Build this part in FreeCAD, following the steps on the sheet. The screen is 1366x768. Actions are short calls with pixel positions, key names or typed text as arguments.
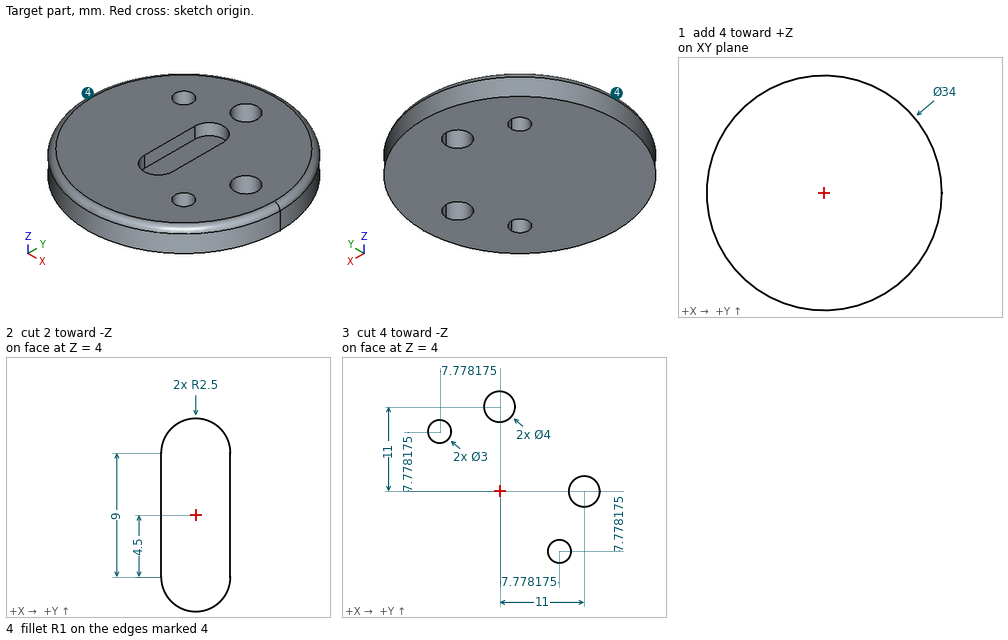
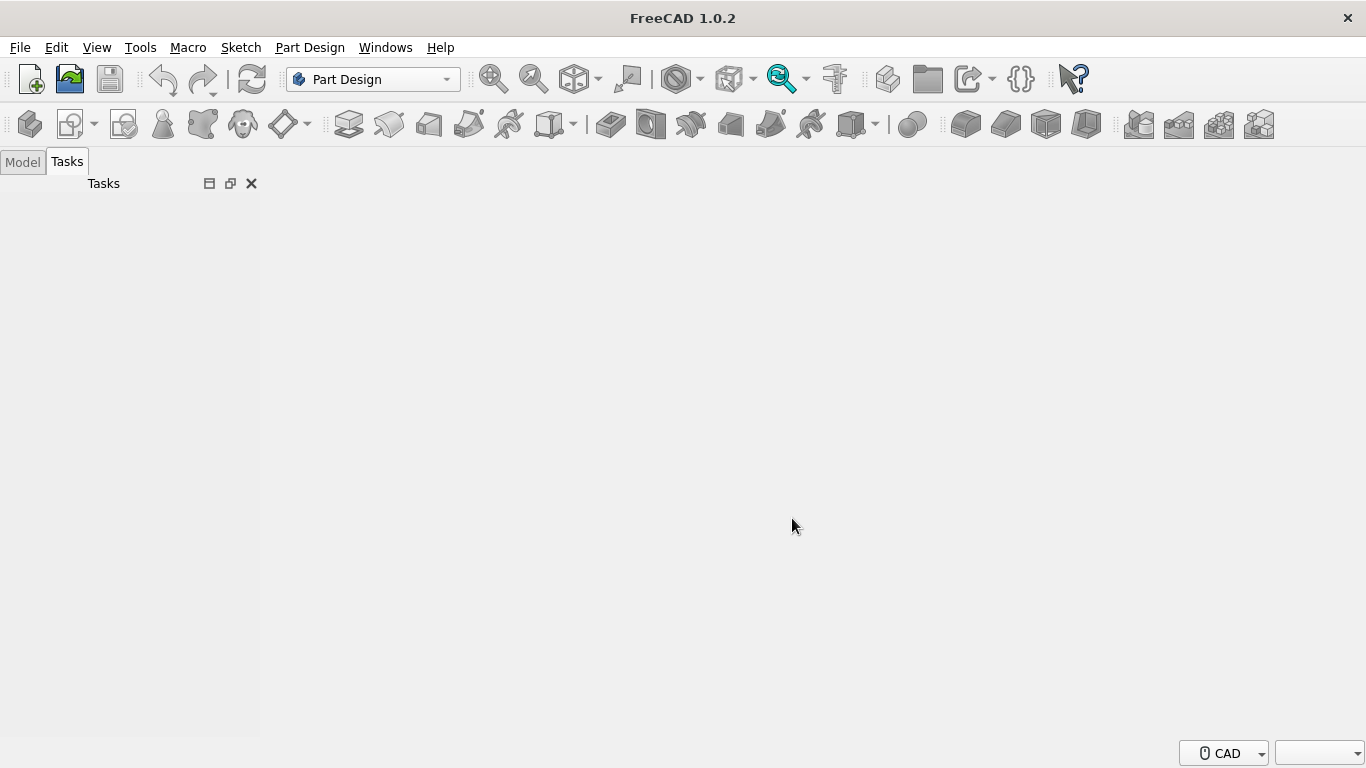
key(ctrl+n)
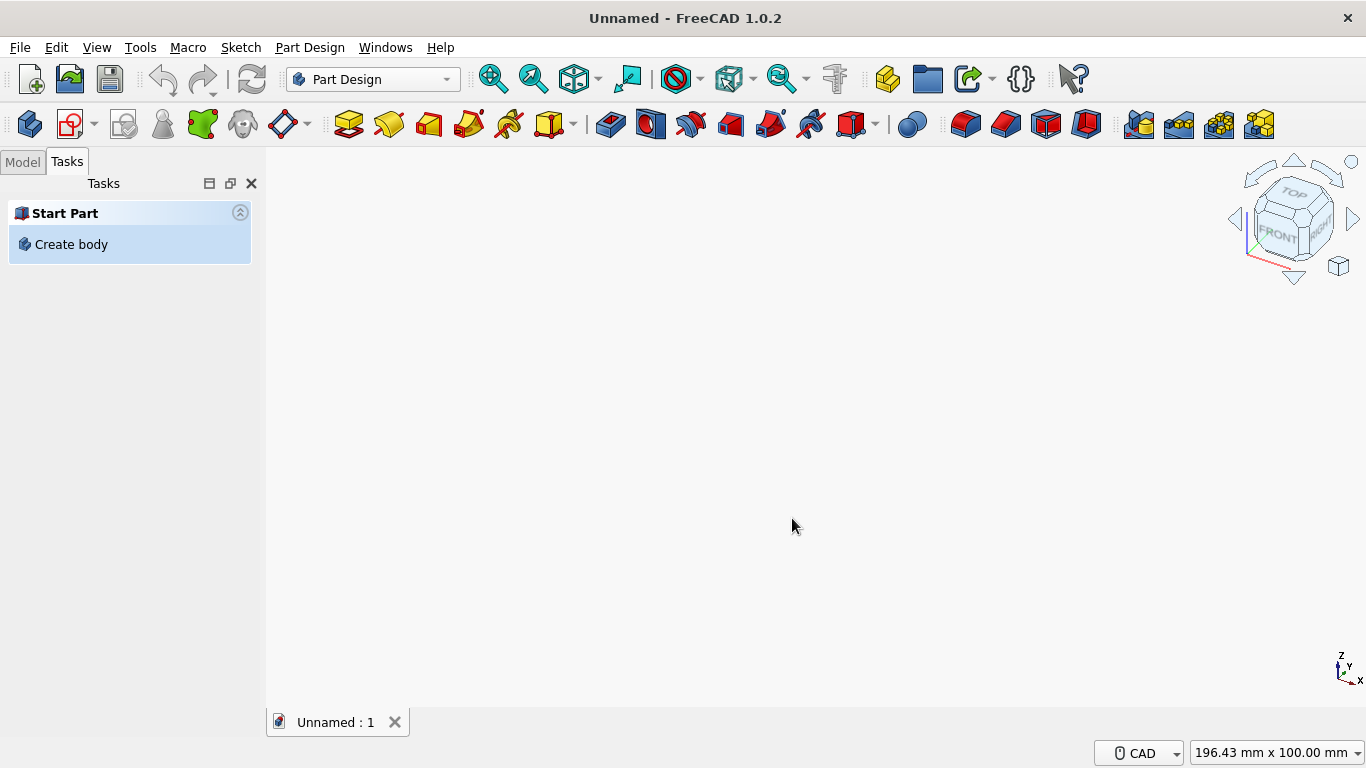
click(70, 124)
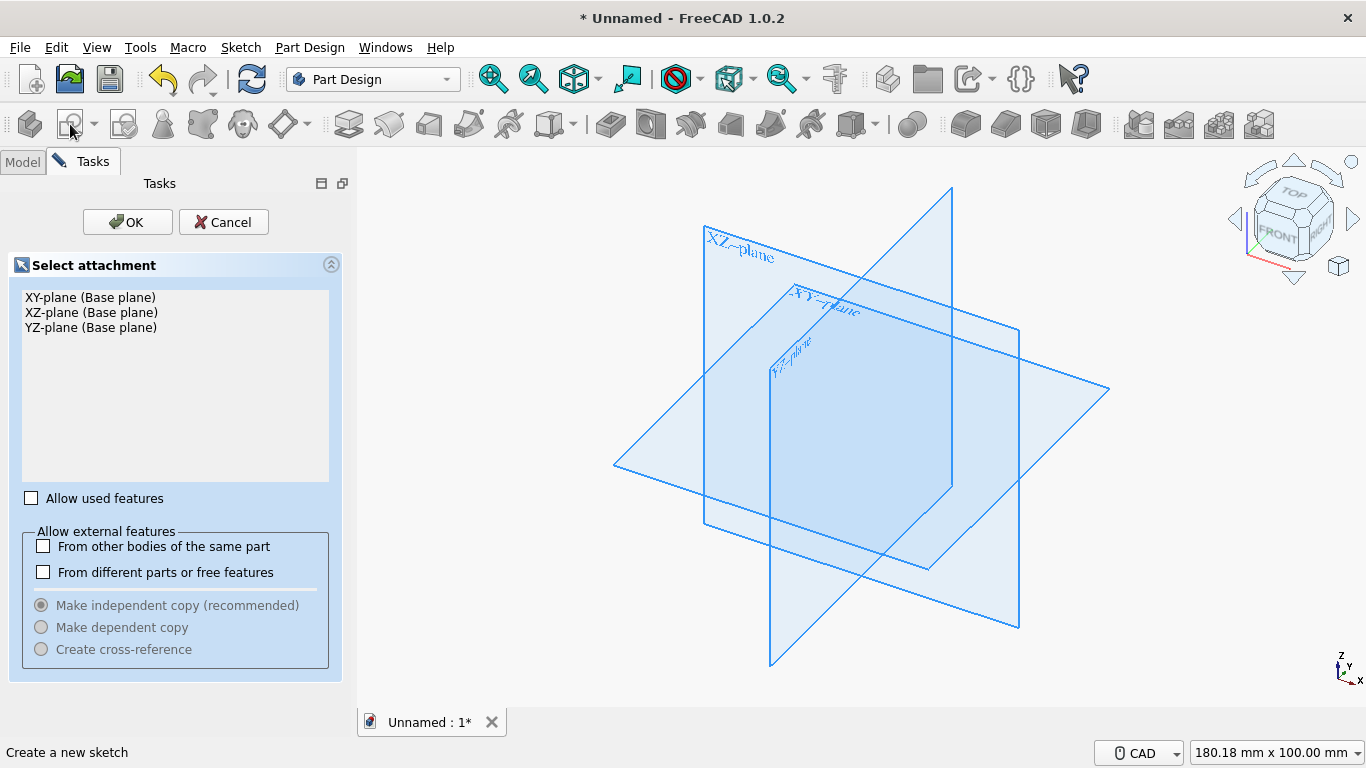
click(82, 298)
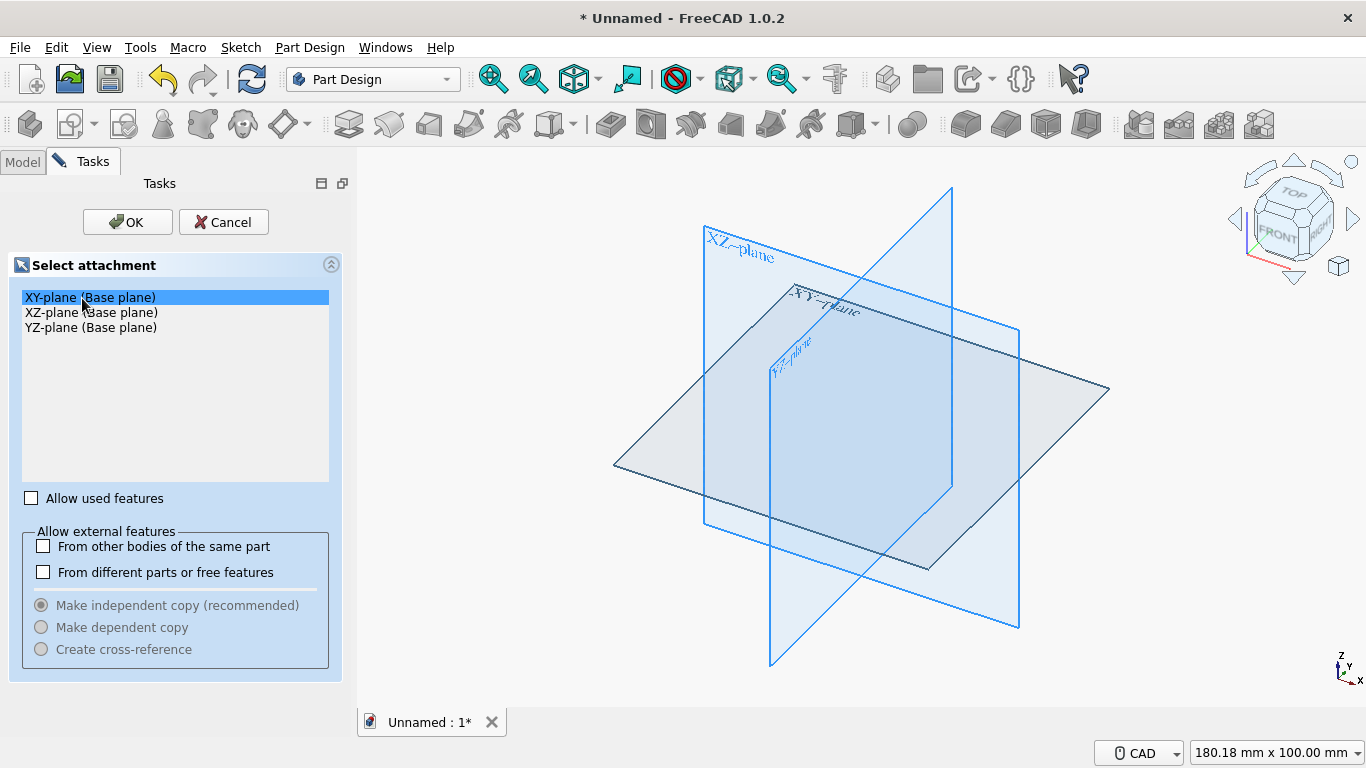
click(128, 222)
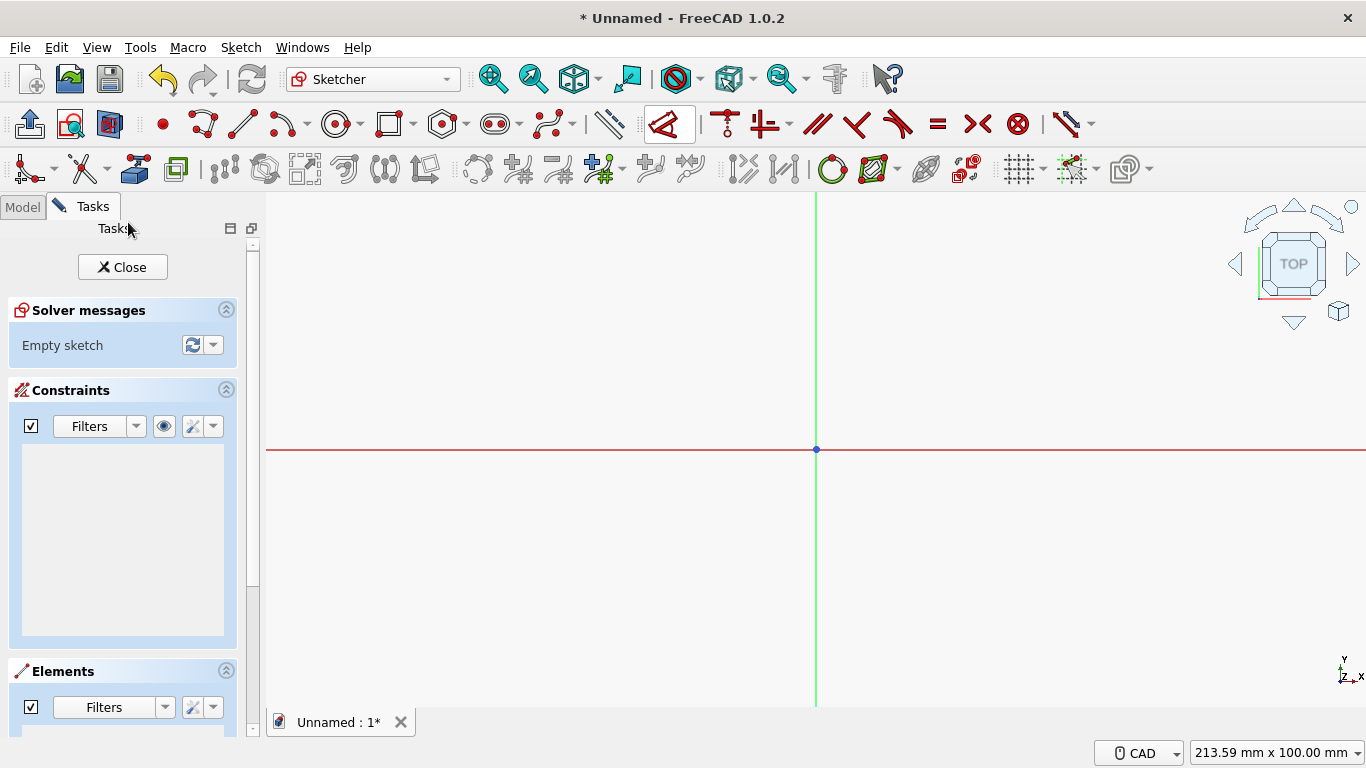
scroll(899, 449, up, 3)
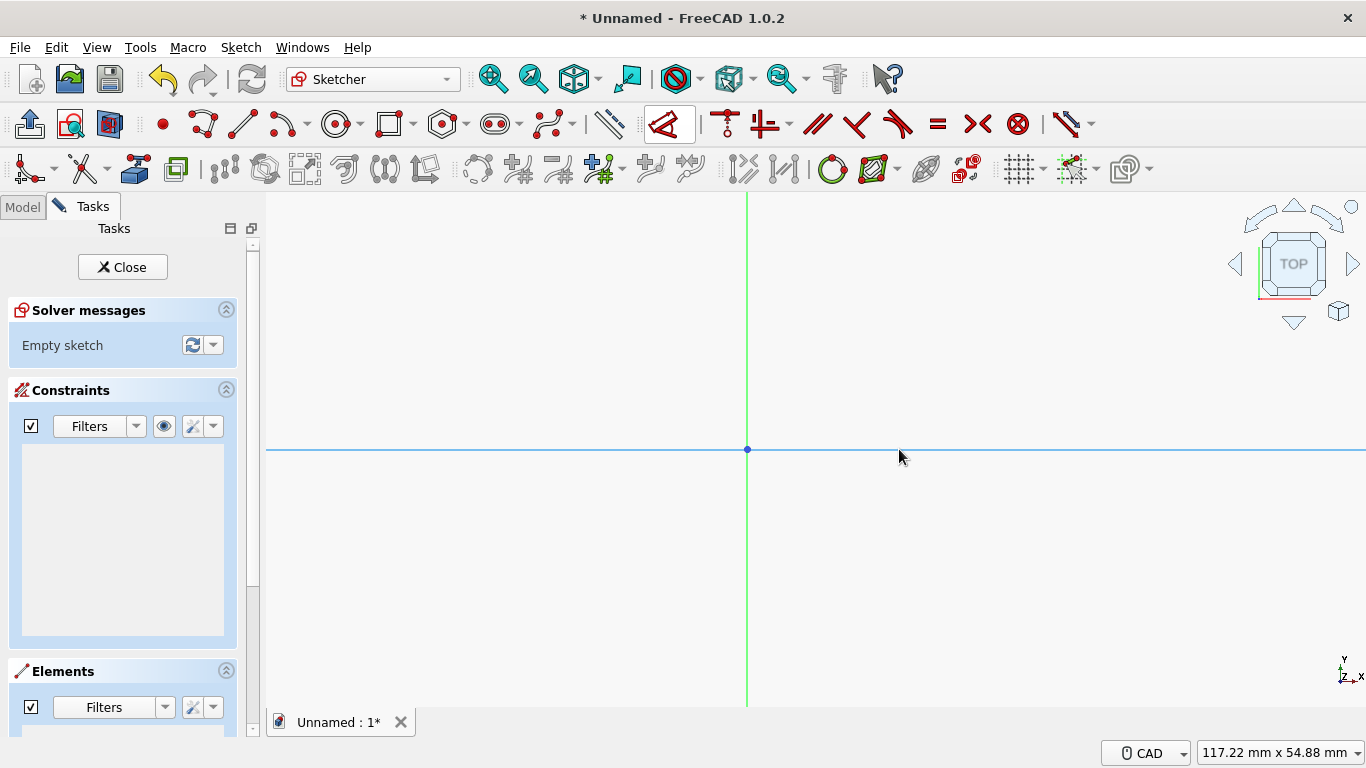
key(g)
key(c)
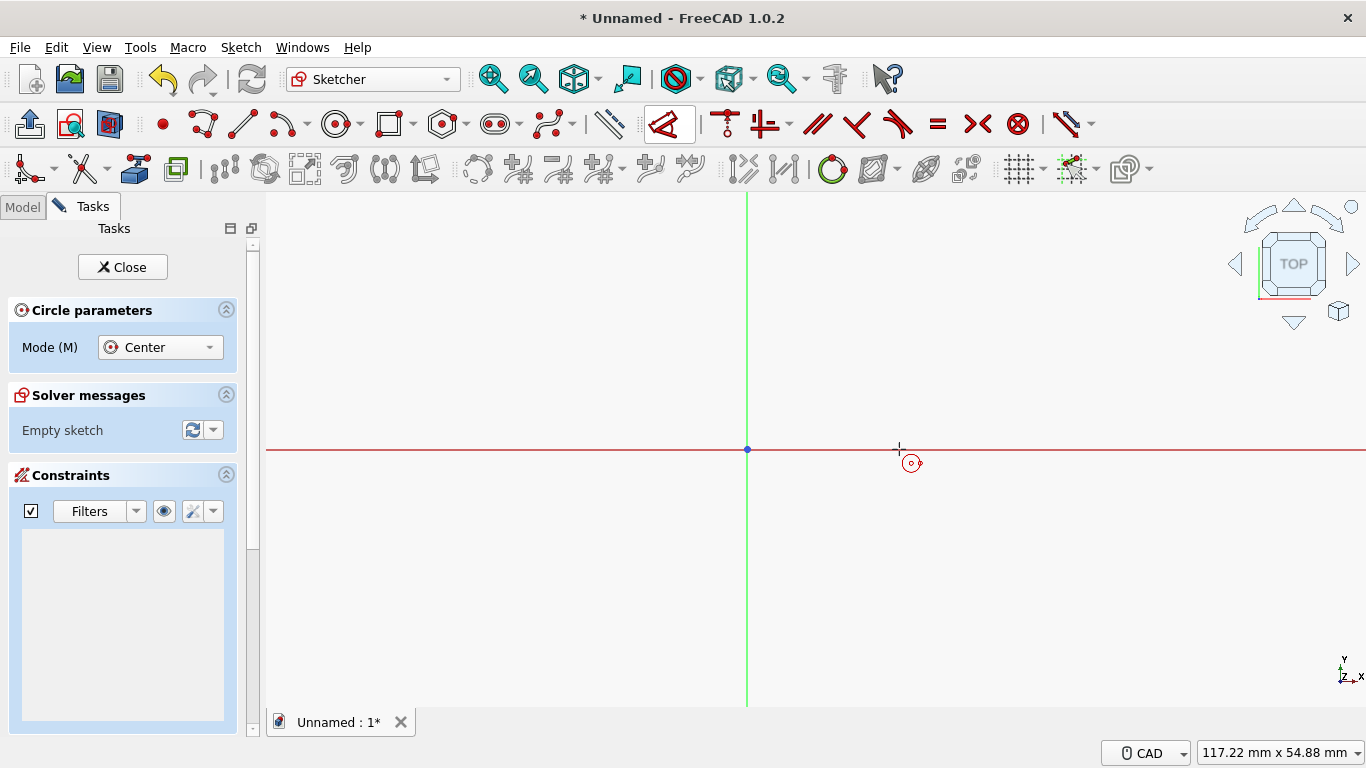
click(747, 450)
click(860, 337)
key(Escape)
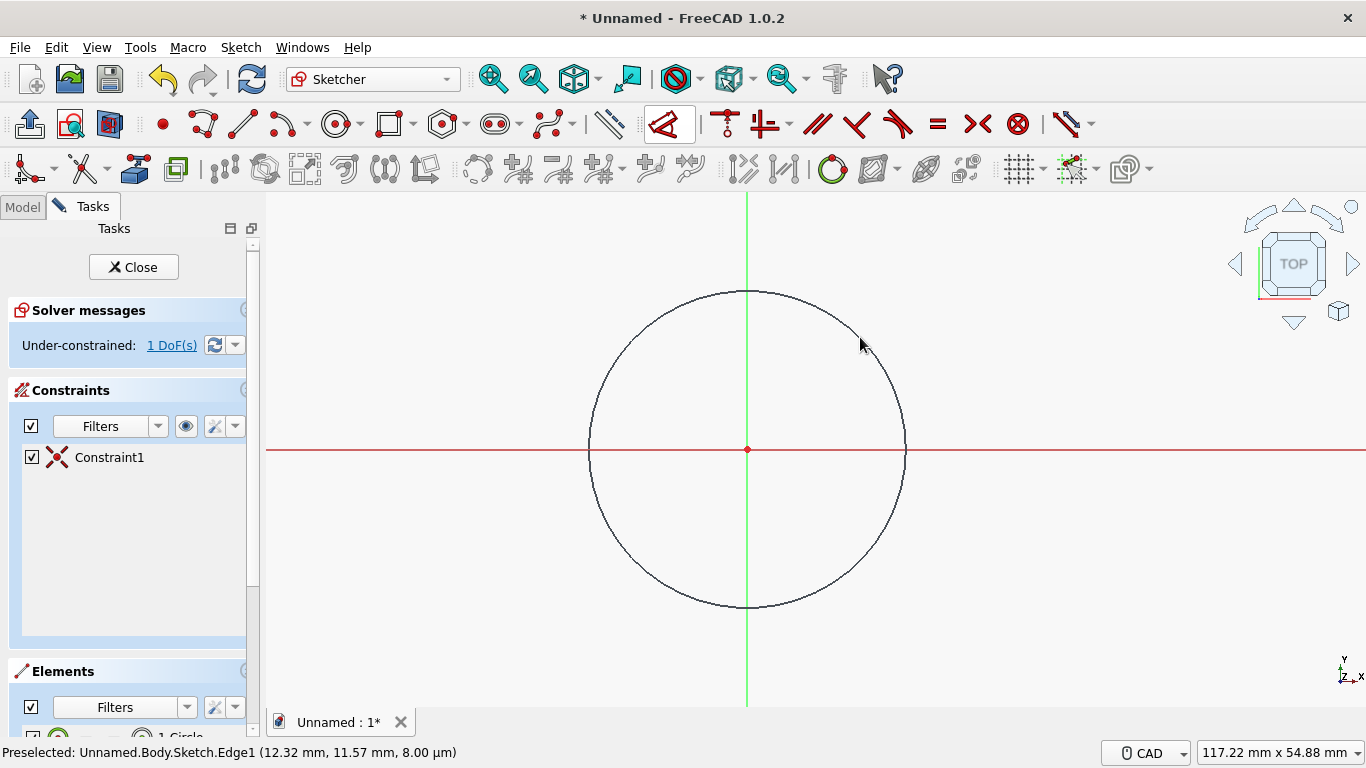
click(664, 124)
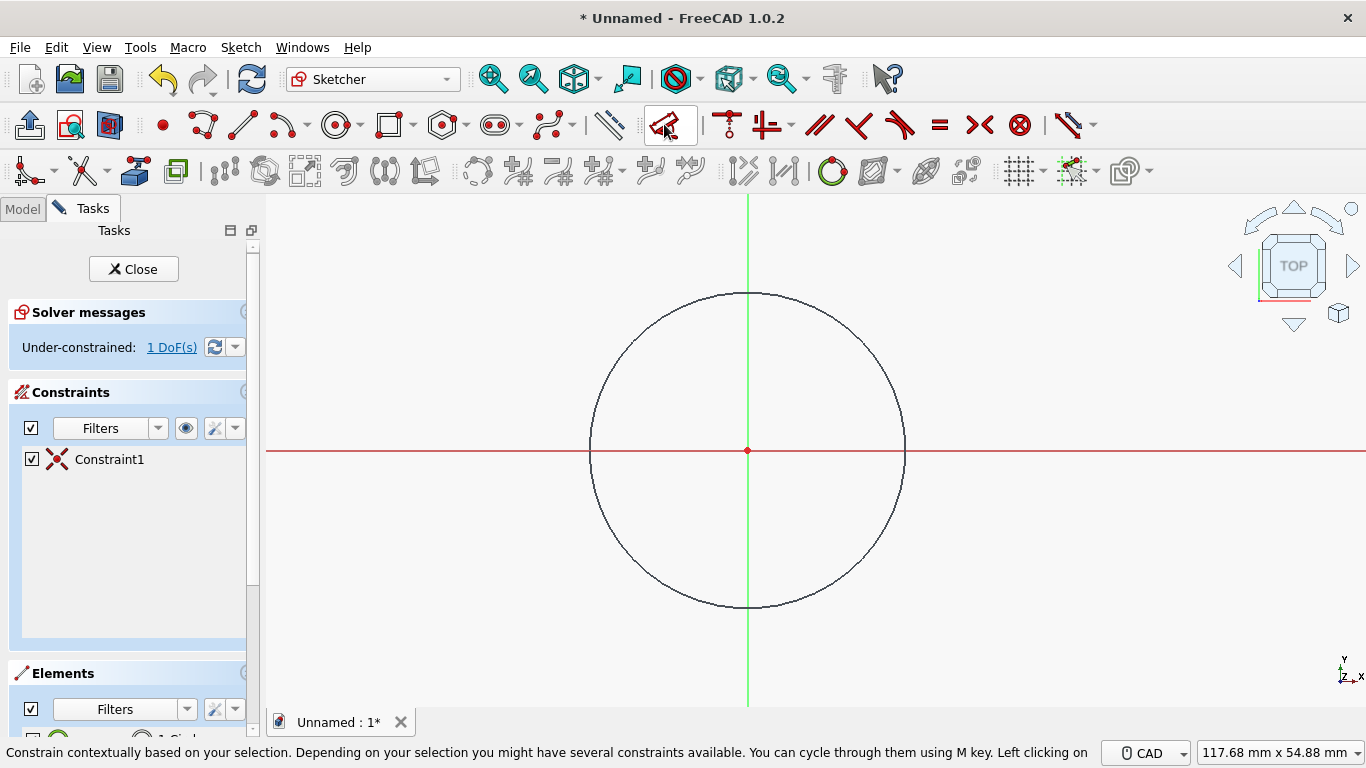
click(859, 338)
click(882, 315)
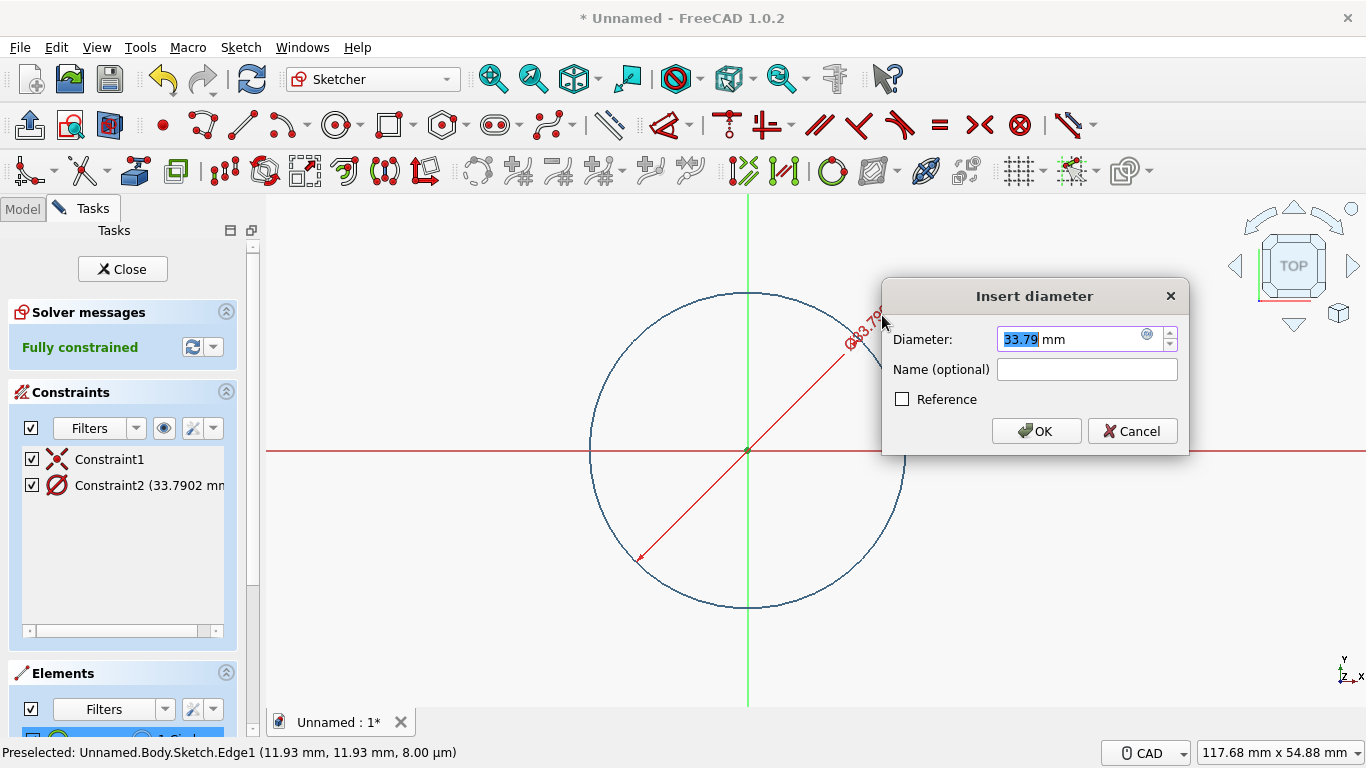
text(34)
key(Return)
key(Escape)